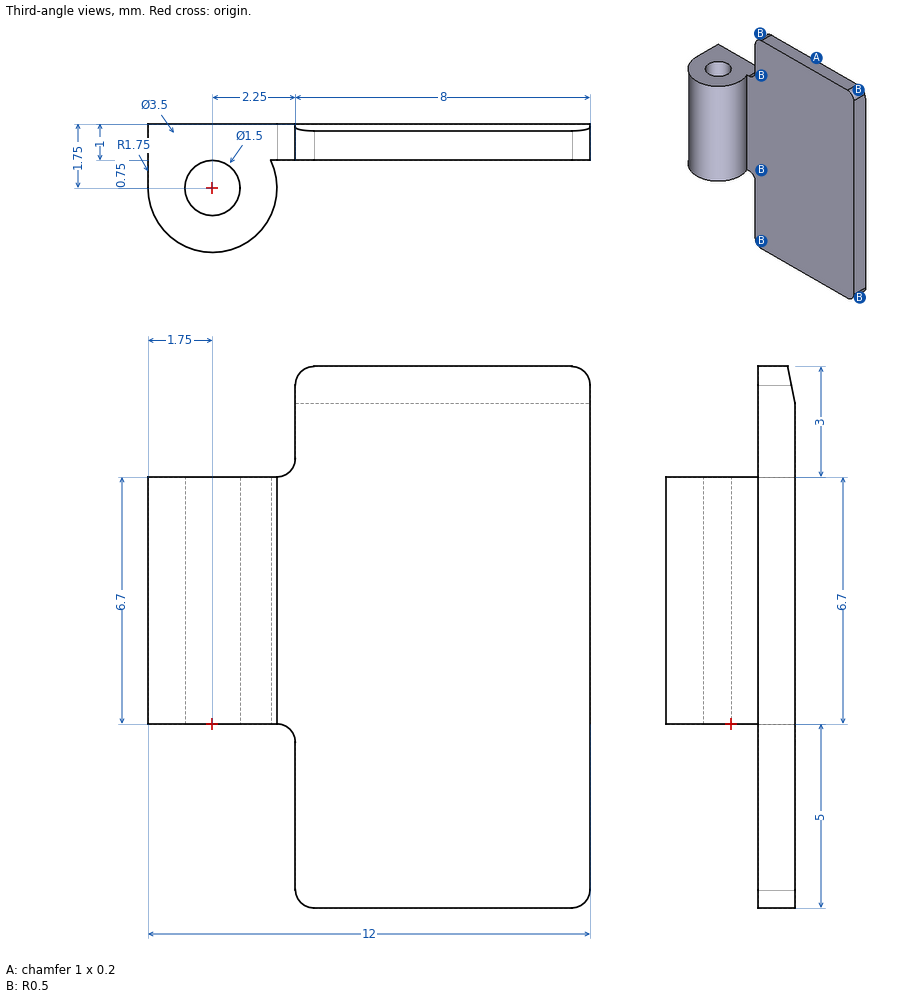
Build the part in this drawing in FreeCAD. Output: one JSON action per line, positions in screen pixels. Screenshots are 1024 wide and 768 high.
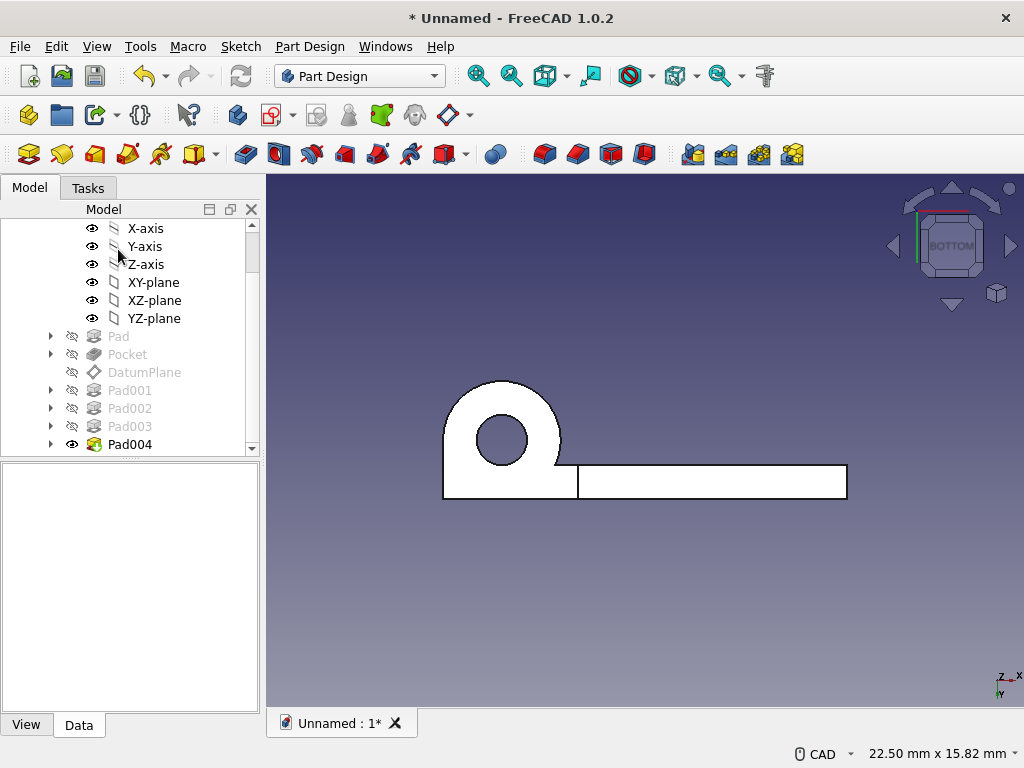
{"action": "key", "text": "0"}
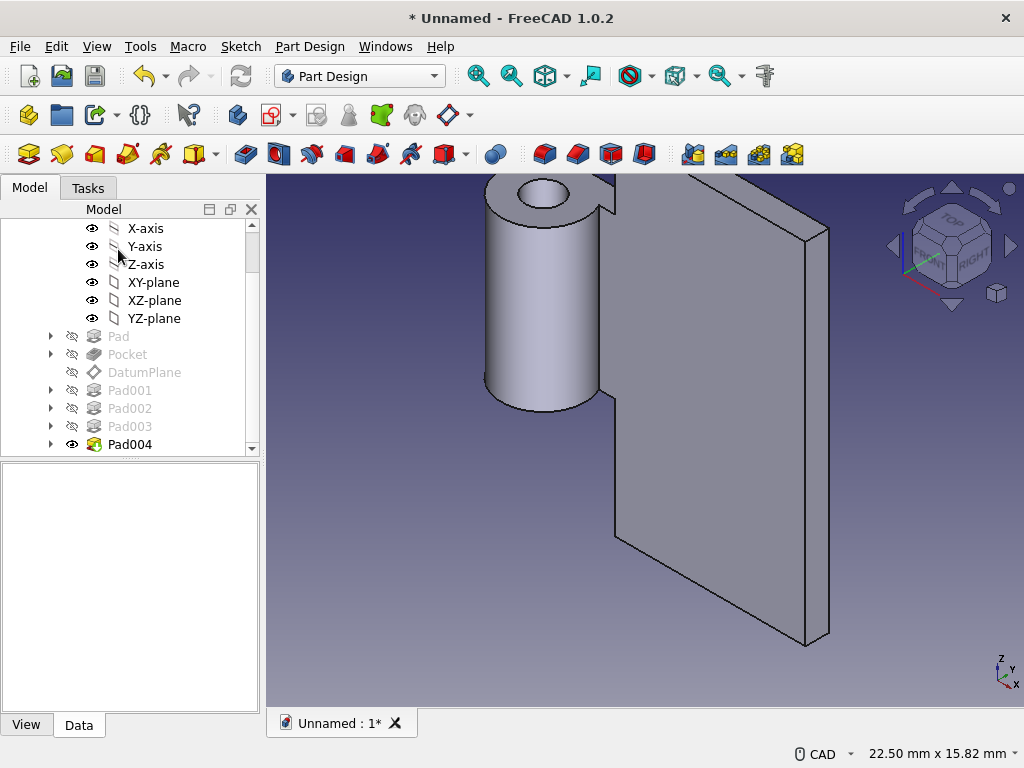
{"action": "left_click", "coordinate": [479, 76]}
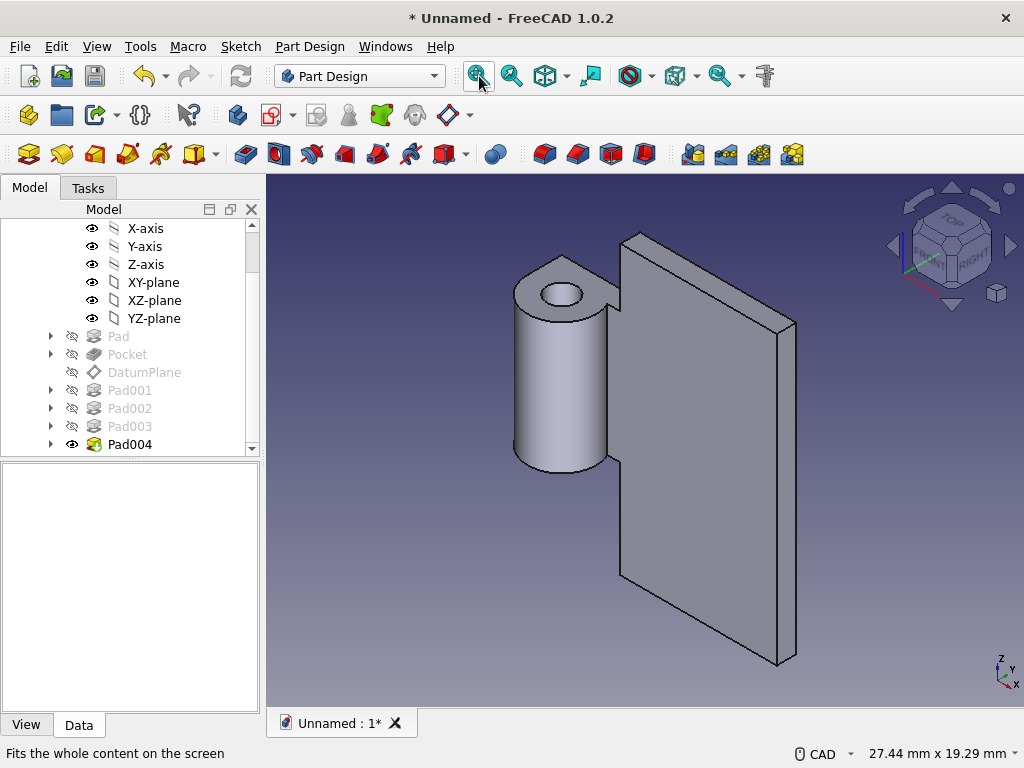
{"action": "key", "text": "2"}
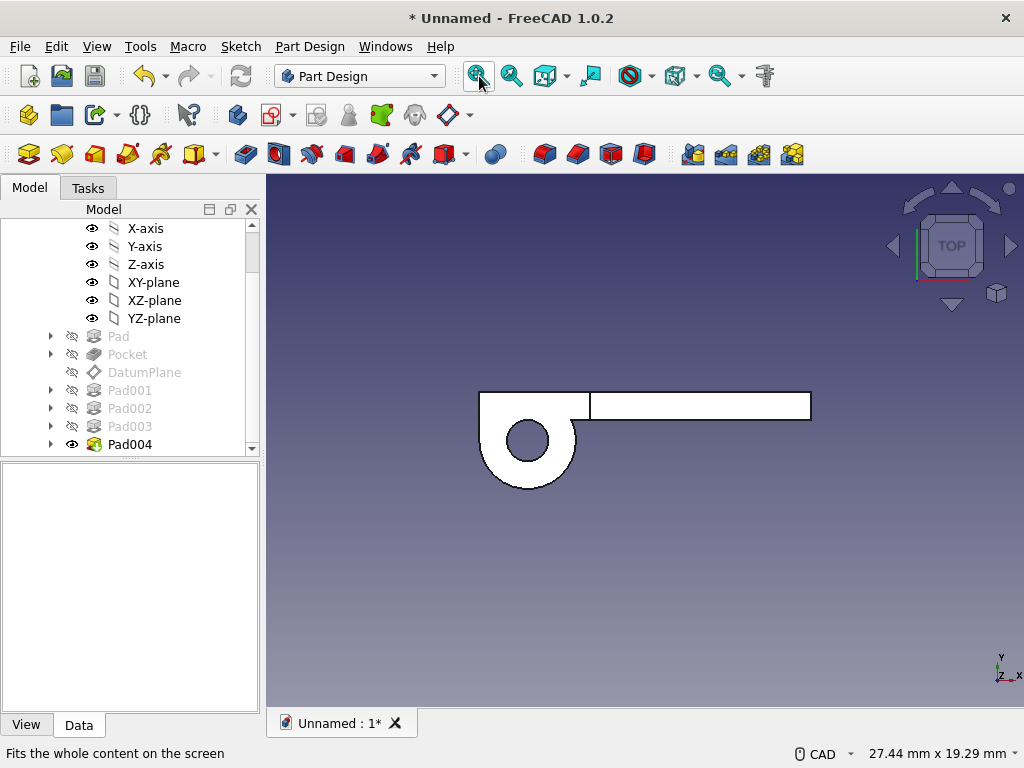
{"action": "left_click", "coordinate": [479, 76]}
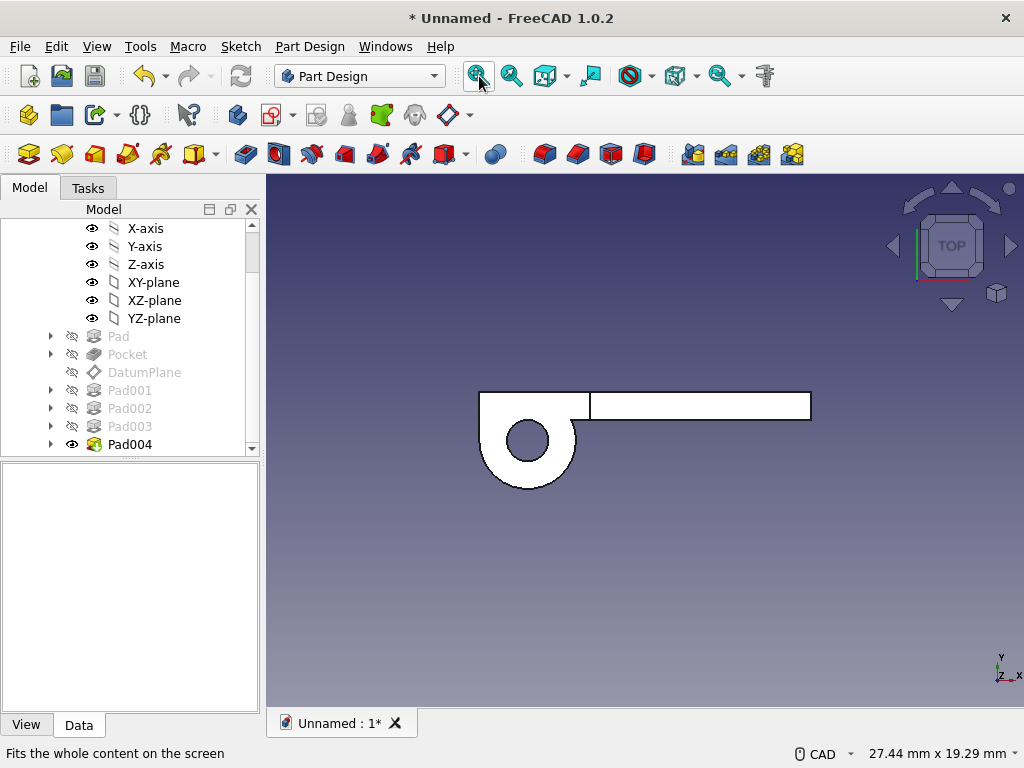
{"action": "left_click", "coordinate": [700, 391]}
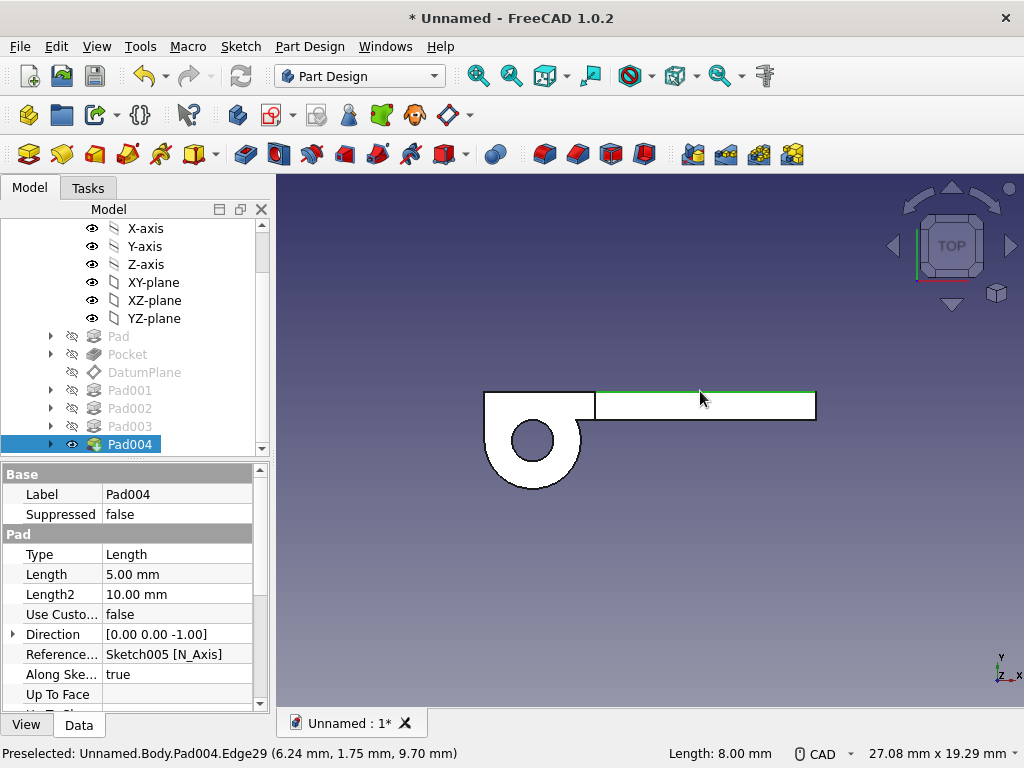
{"action": "left_click", "coordinate": [578, 154]}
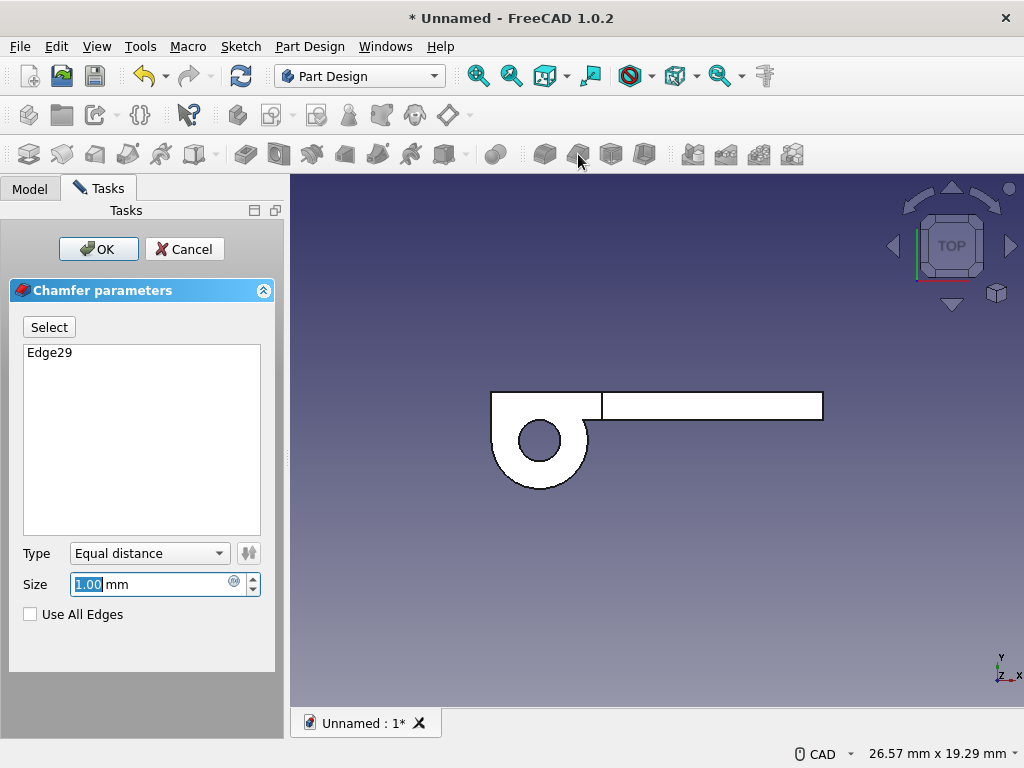
{"action": "type", "text": "1"}
{"action": "key", "text": "Tab"}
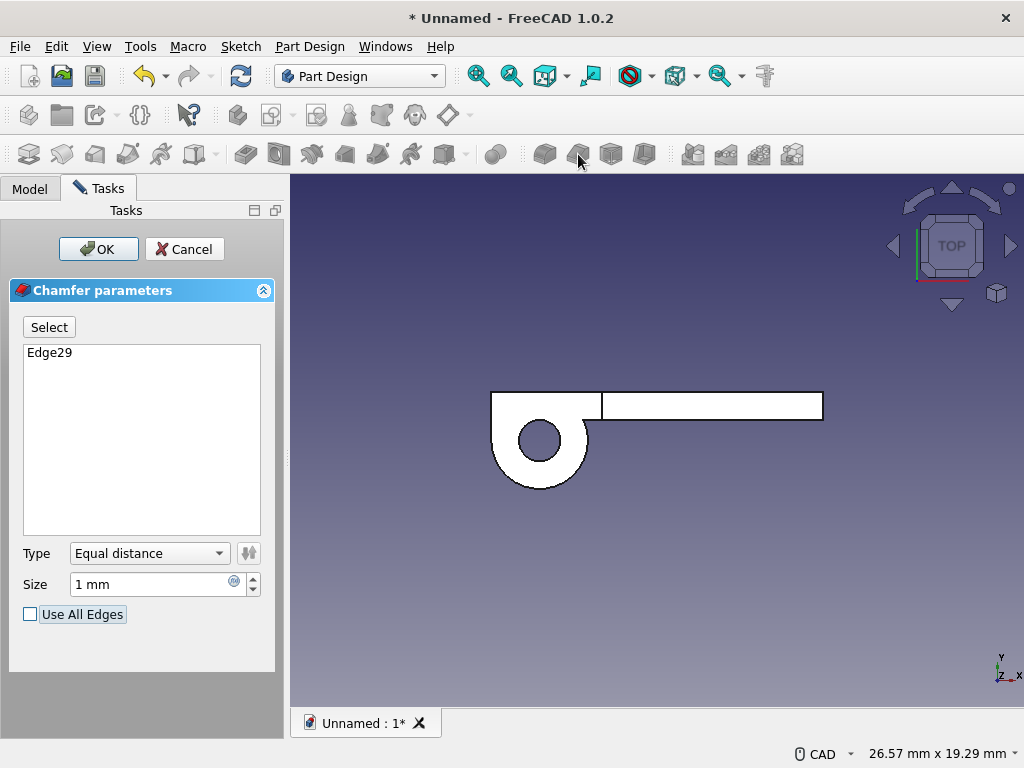
{"action": "left_click", "coordinate": [150, 554]}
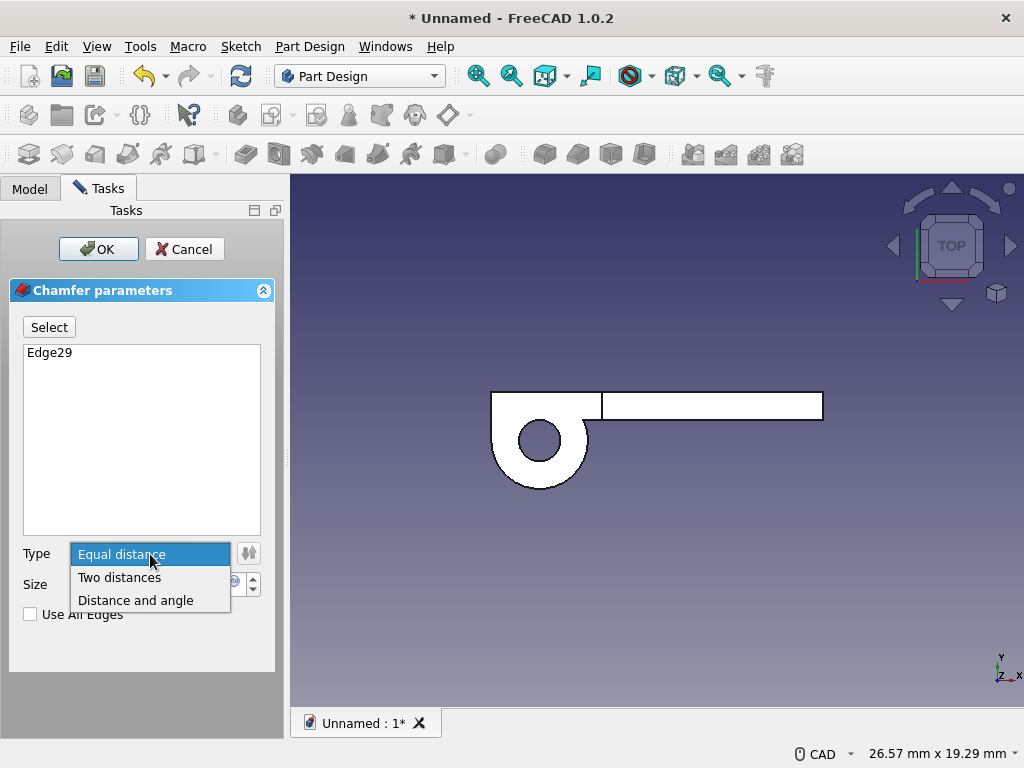
{"action": "left_click", "coordinate": [148, 578]}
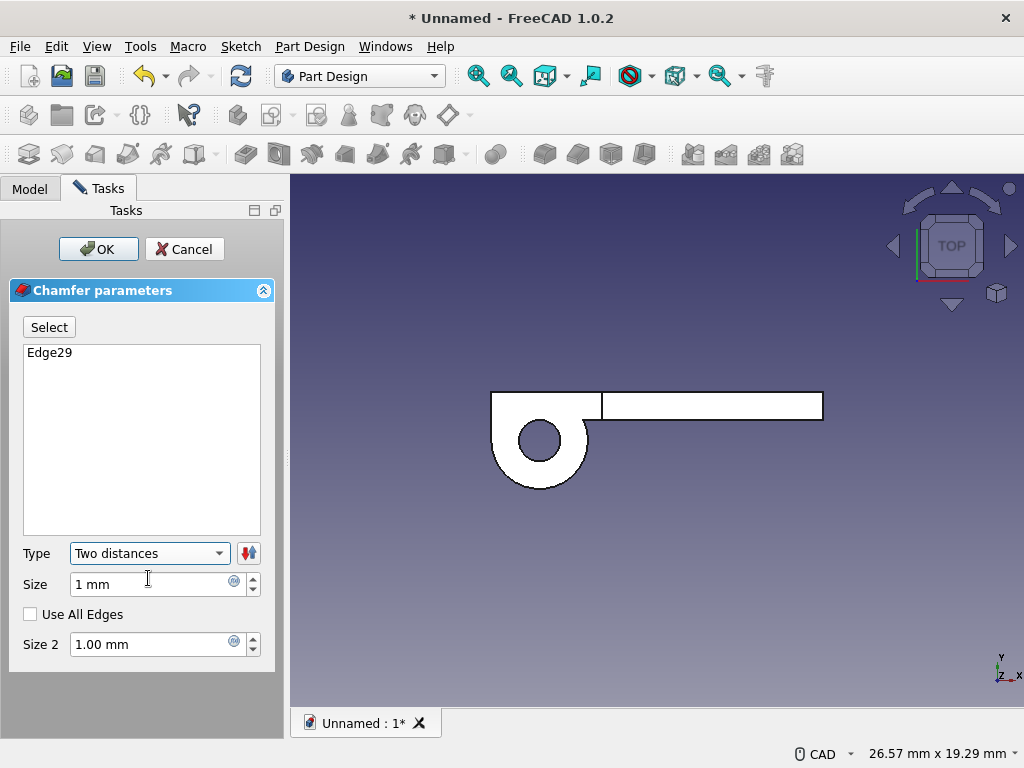
{"action": "triple_click", "coordinate": [158, 644]}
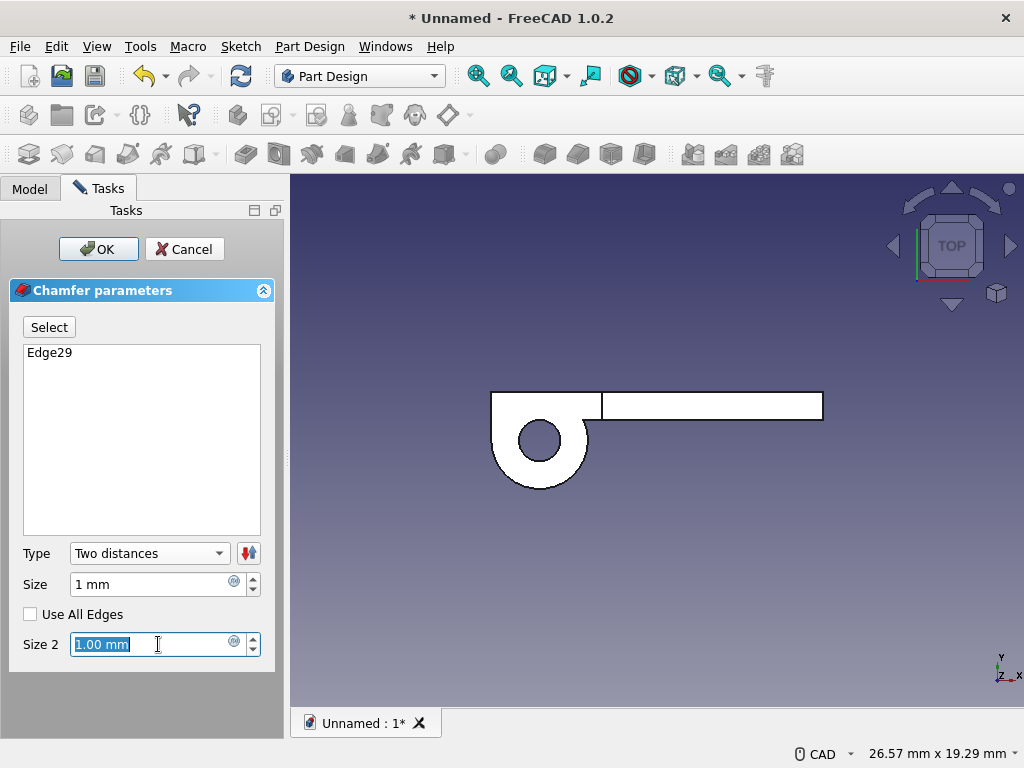
{"action": "type", "text": "0.2"}
{"action": "key", "text": "Tab"}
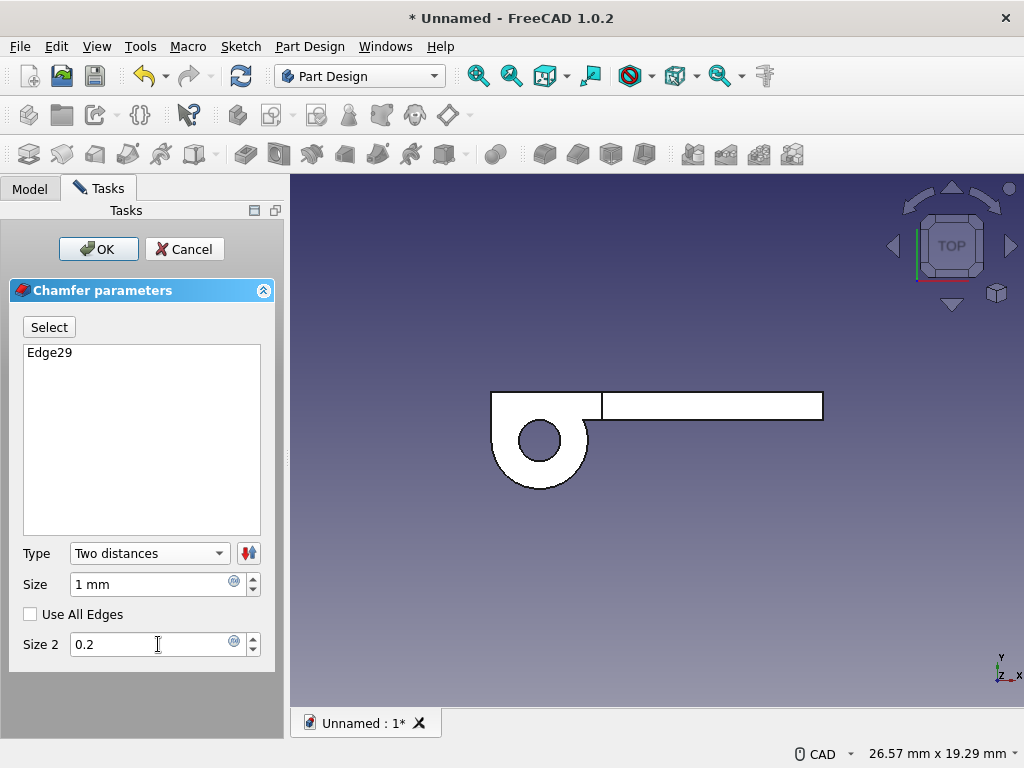
{"action": "left_click", "coordinate": [249, 554]}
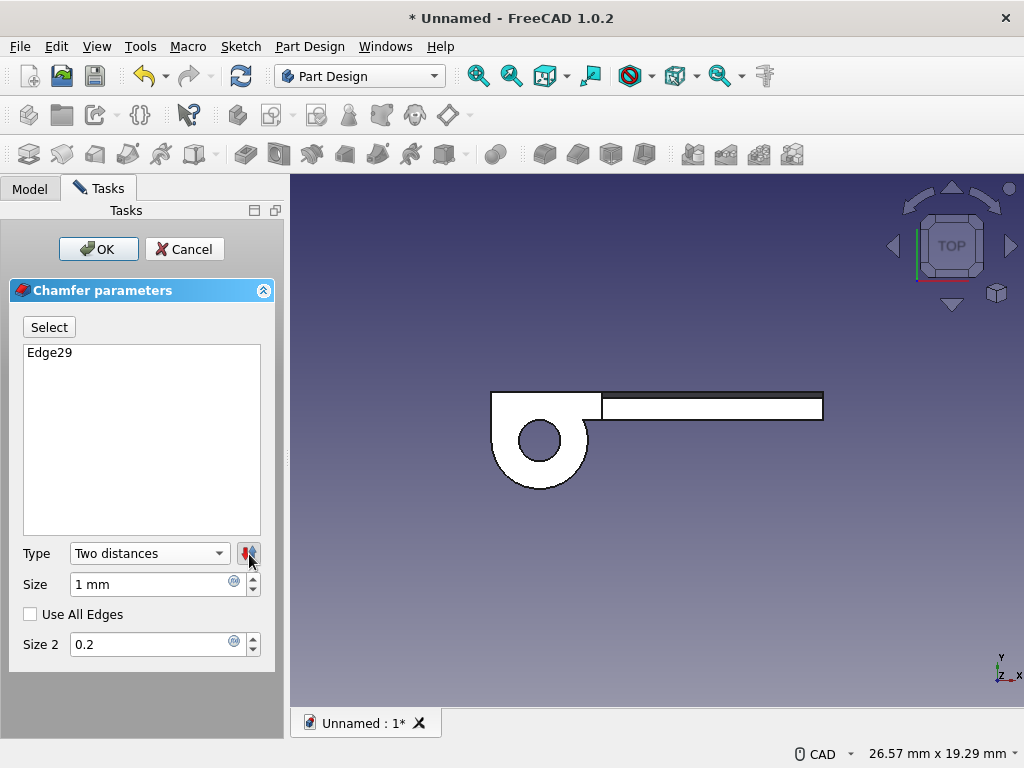
{"action": "left_click", "coordinate": [99, 249]}